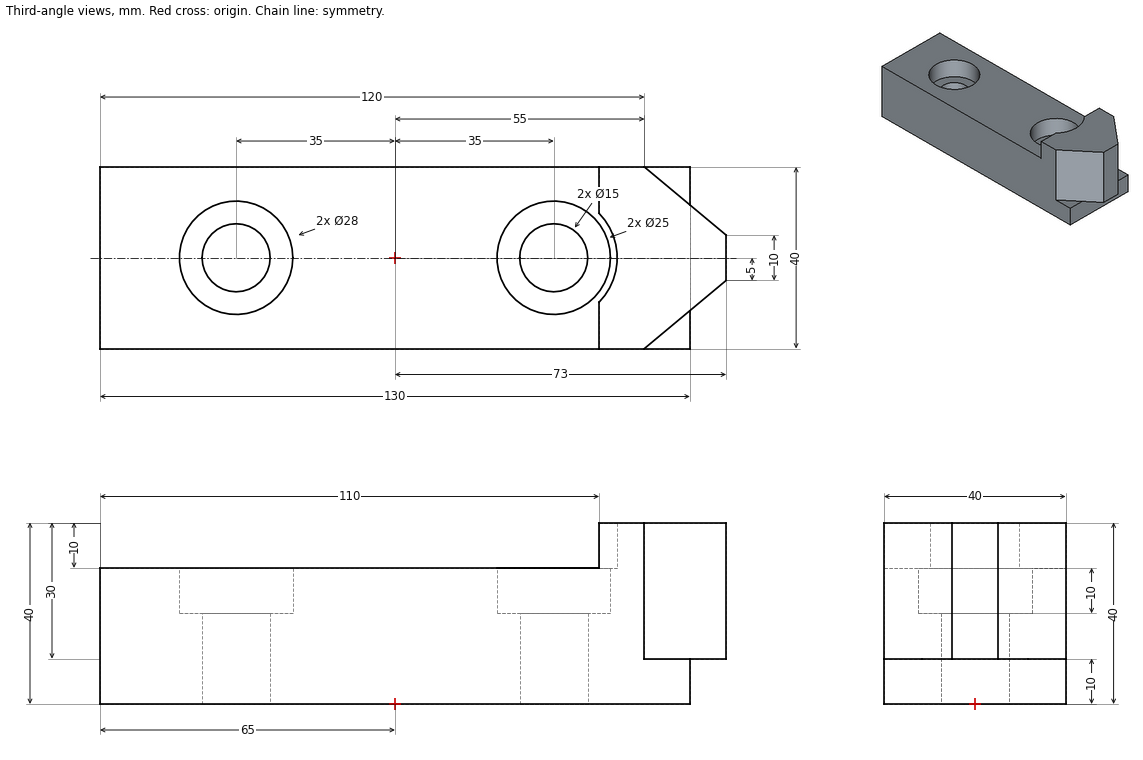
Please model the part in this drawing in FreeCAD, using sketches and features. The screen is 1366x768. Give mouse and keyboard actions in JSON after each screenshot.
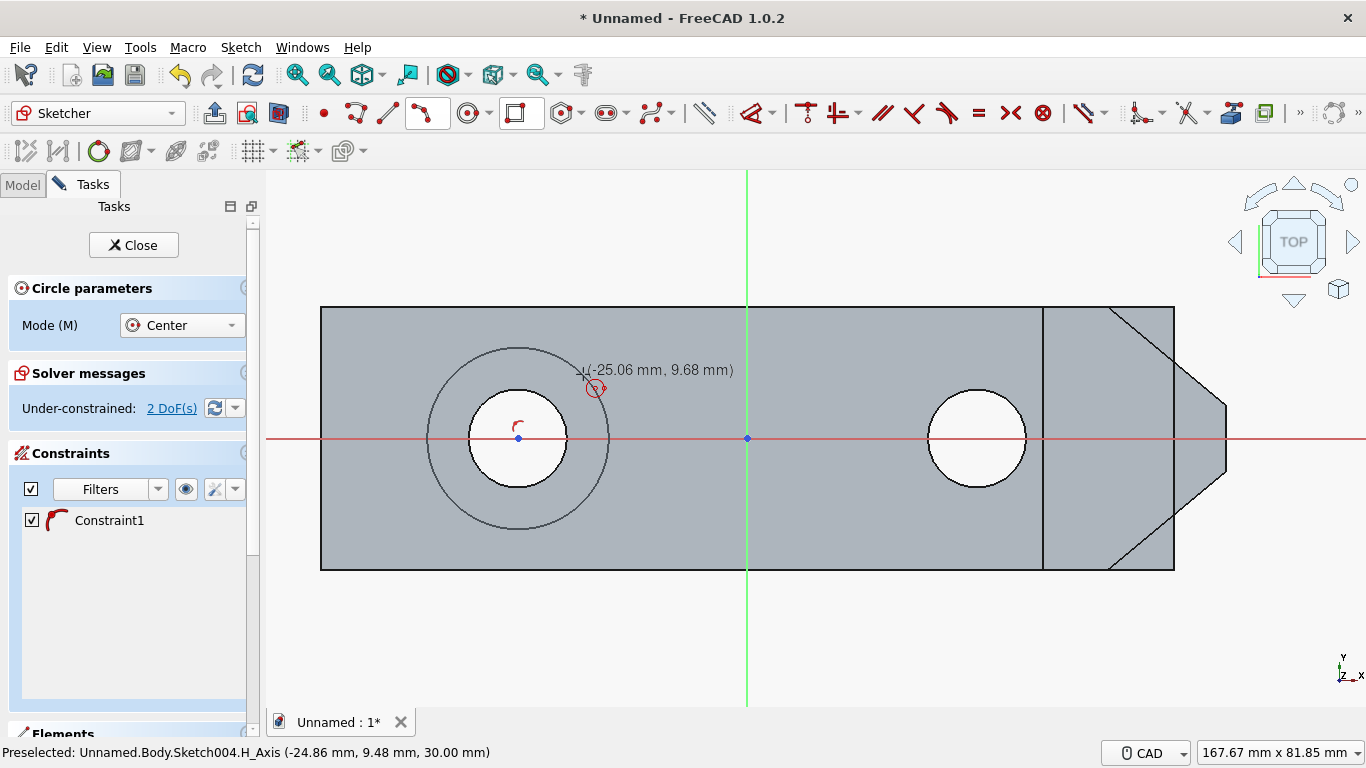
{"action": "left_click", "coordinate": [977, 438]}
{"action": "left_click", "coordinate": [1042, 374]}
{"action": "key", "text": "Escape"}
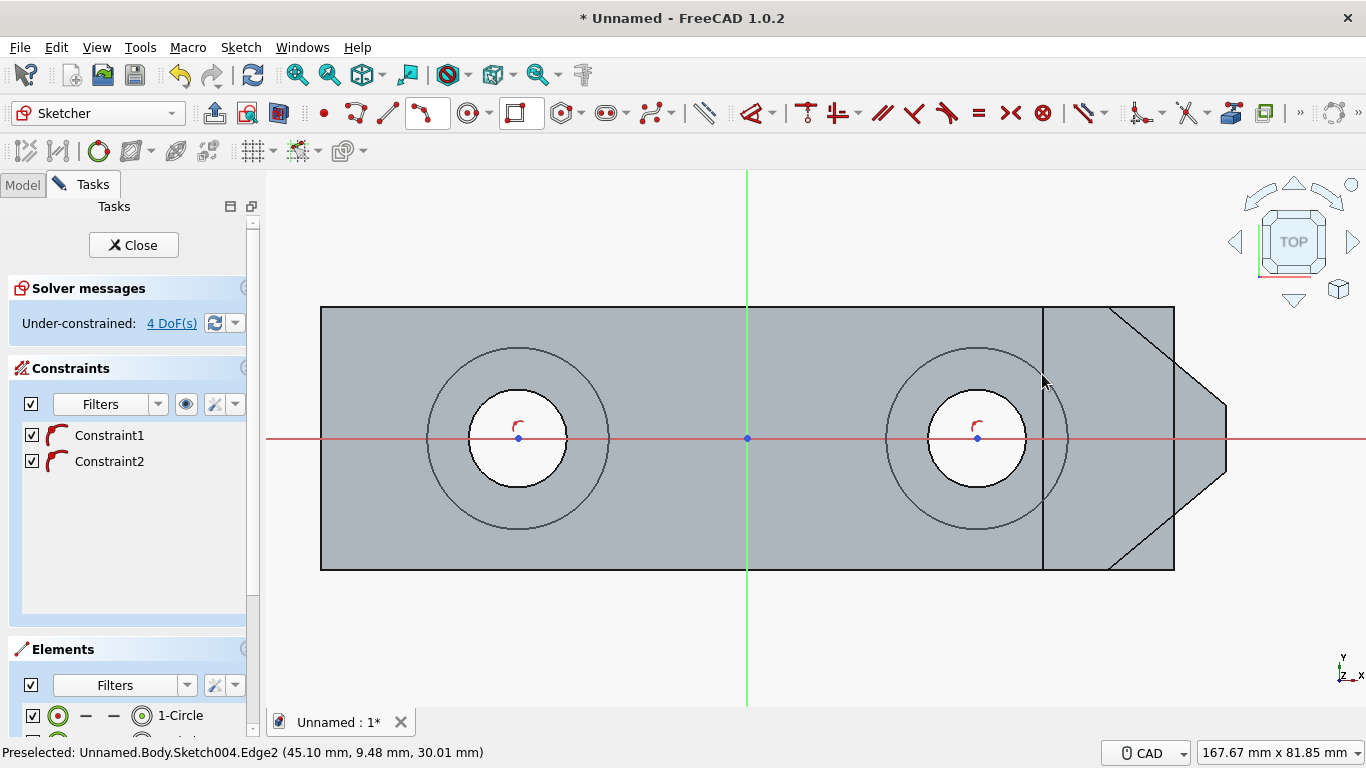
{"action": "left_click", "coordinate": [582, 374]}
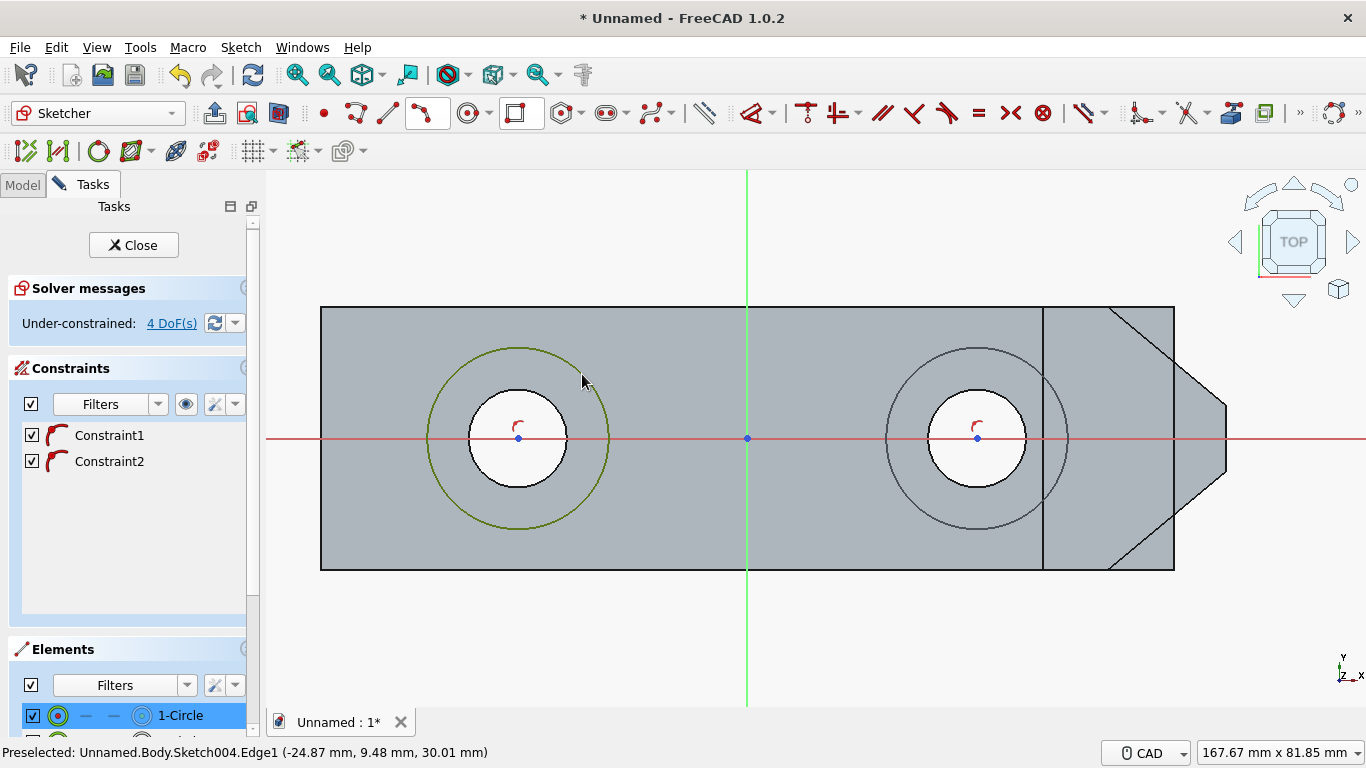
{"action": "left_click", "coordinate": [1041, 374]}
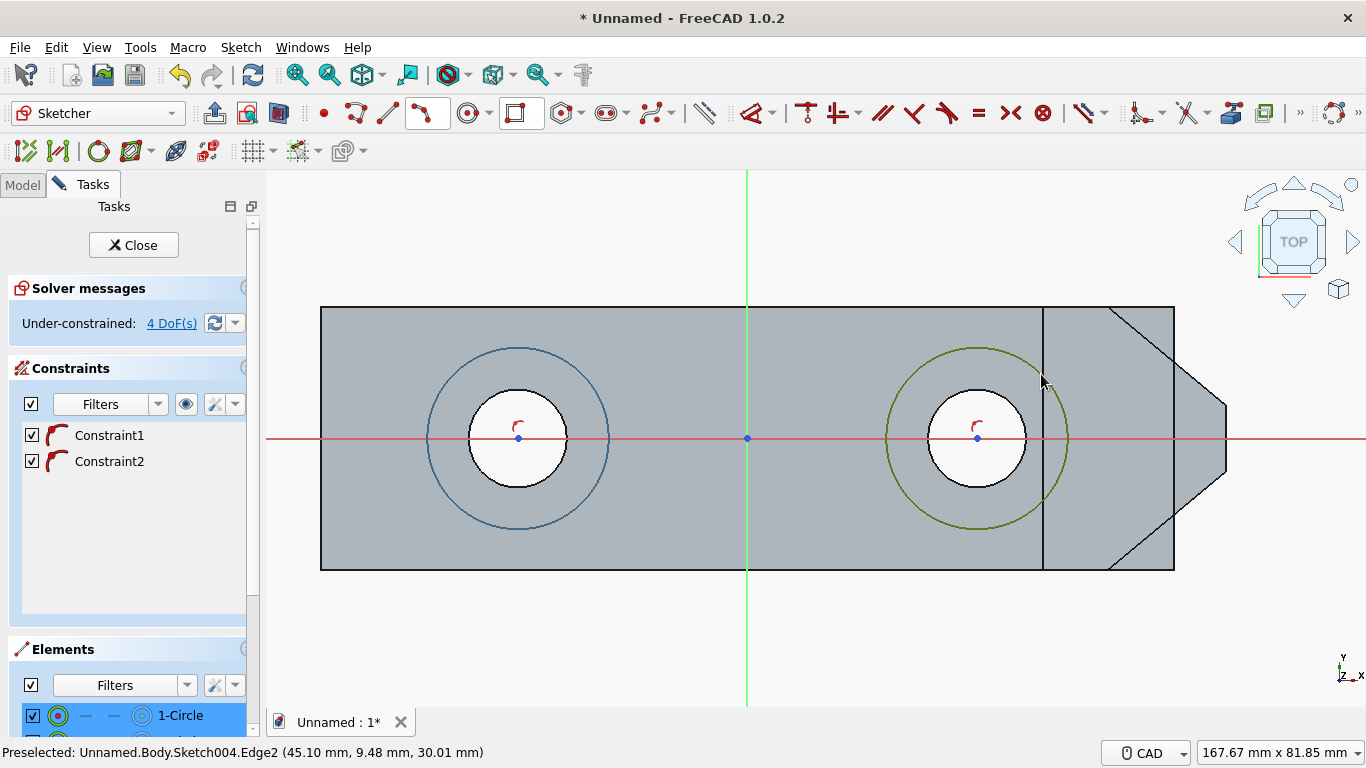
{"action": "key", "text": "e"}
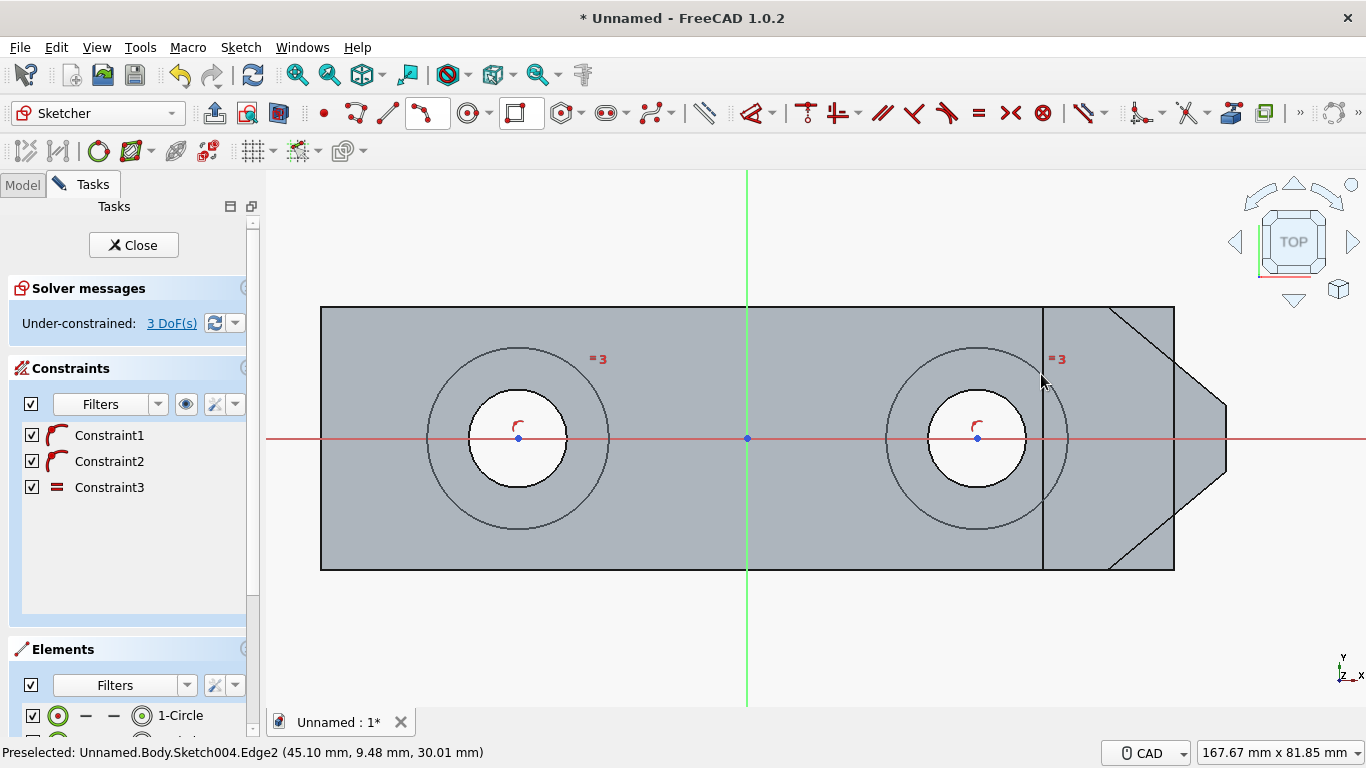
{"action": "left_click", "coordinate": [752, 114]}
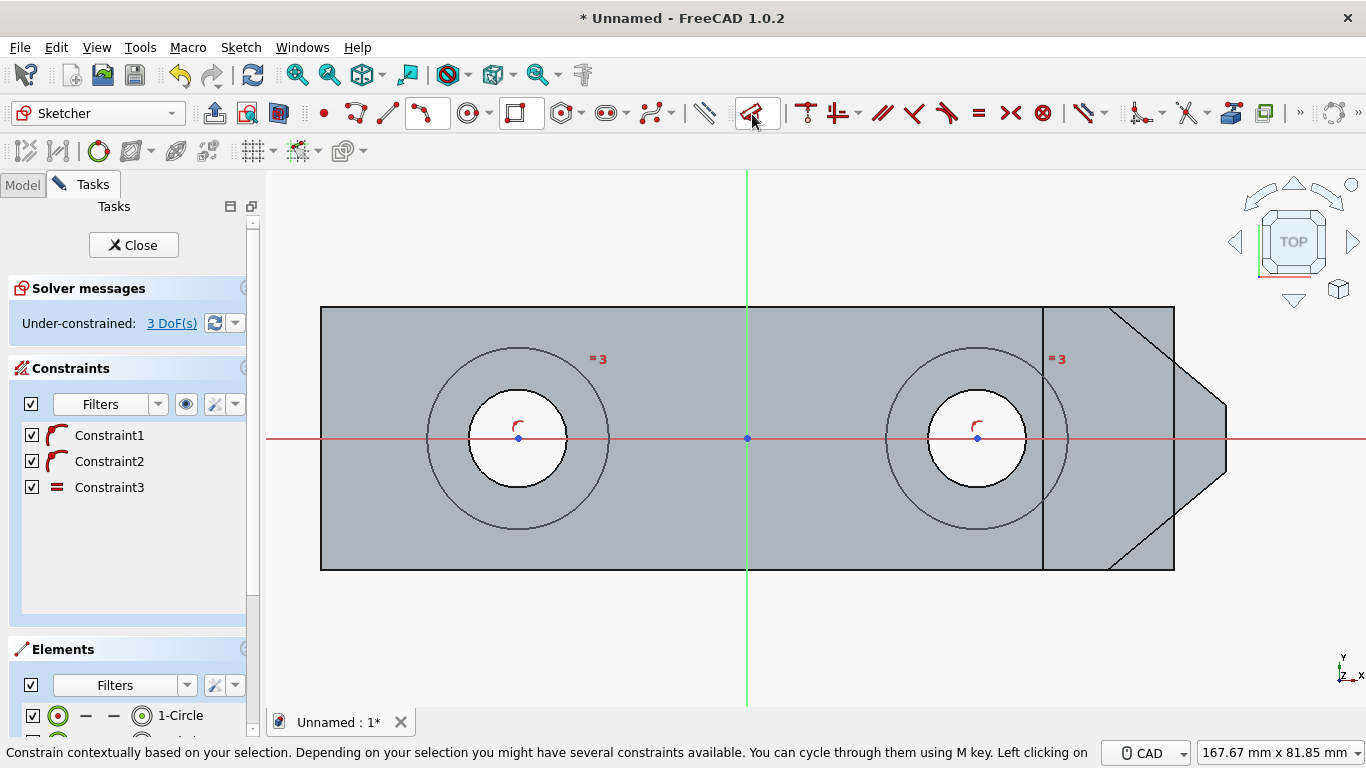
{"action": "left_click", "coordinate": [582, 374]}
{"action": "left_click", "coordinate": [605, 351]}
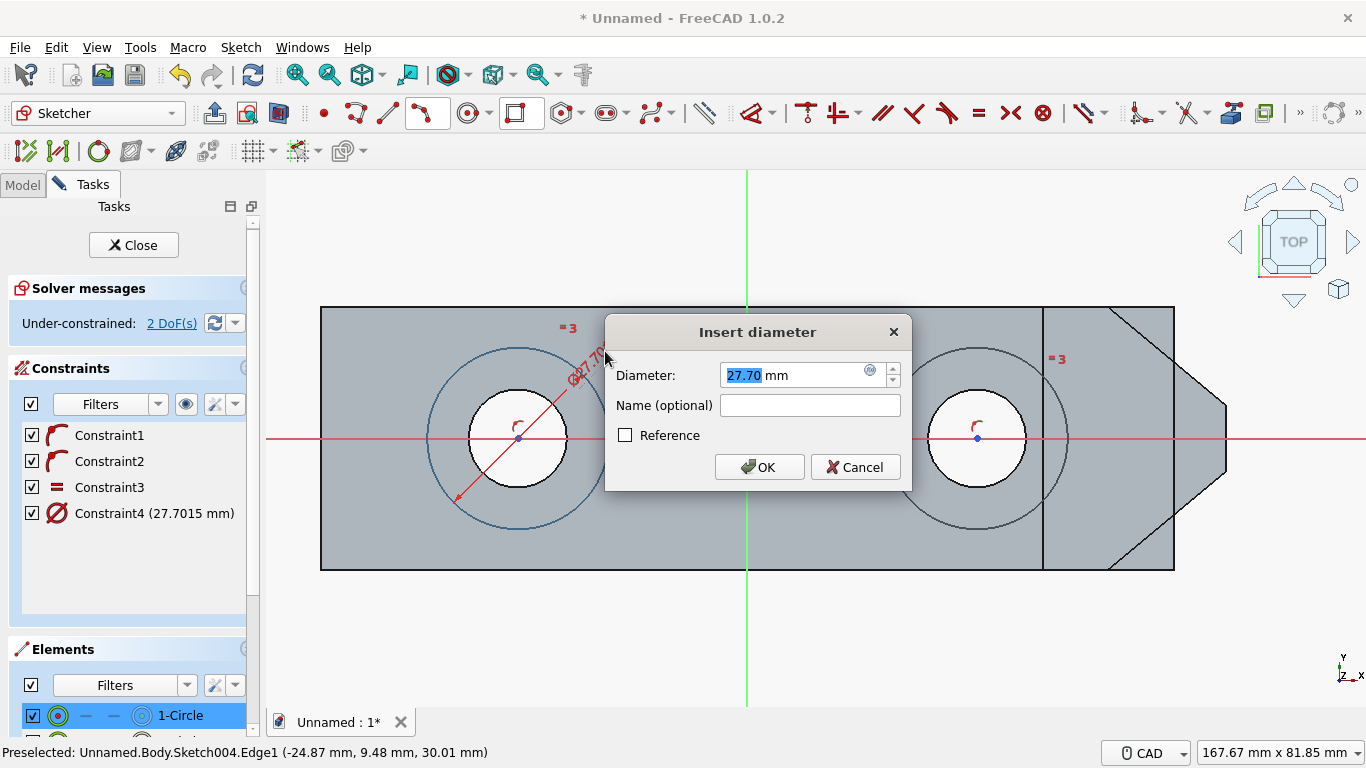
{"action": "type", "text": "28"}
{"action": "key", "text": "Return"}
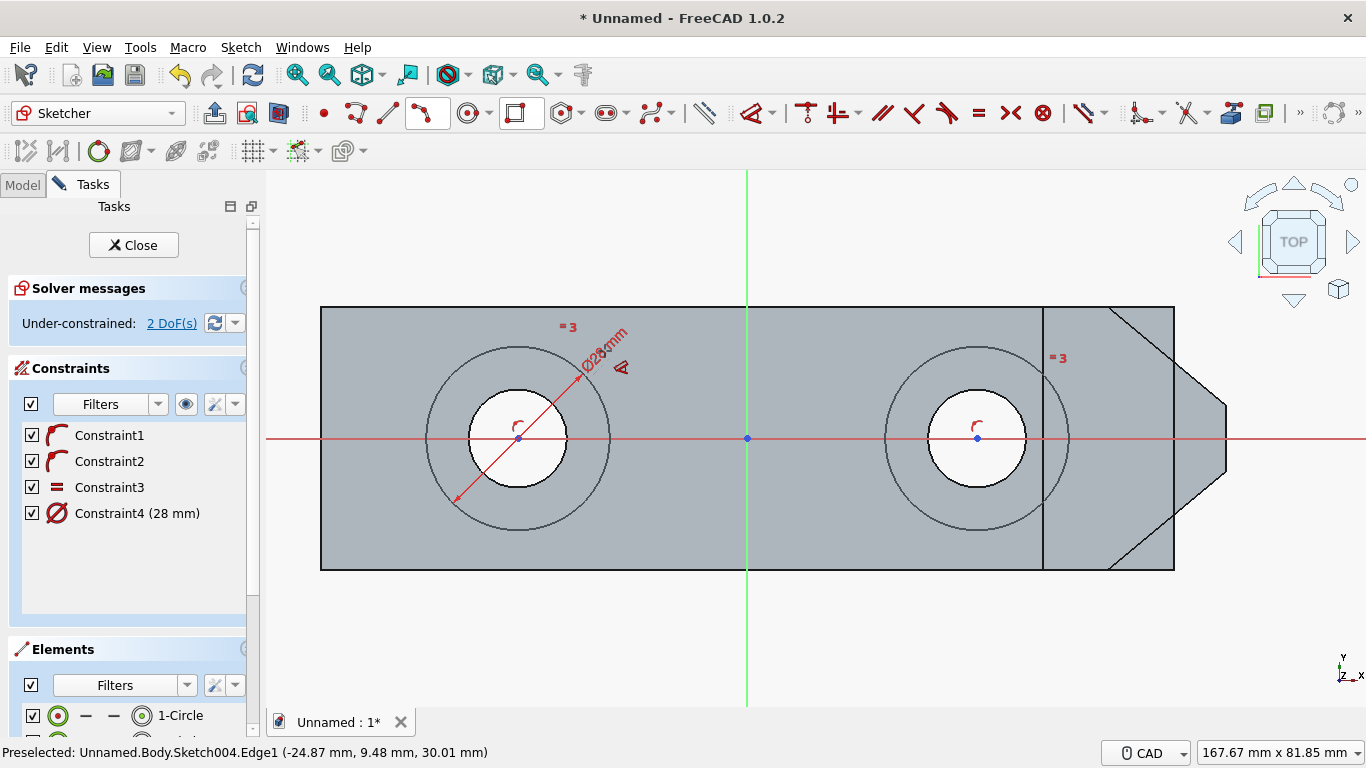
{"action": "left_click", "coordinate": [518, 438]}
{"action": "left_click", "coordinate": [633, 472]}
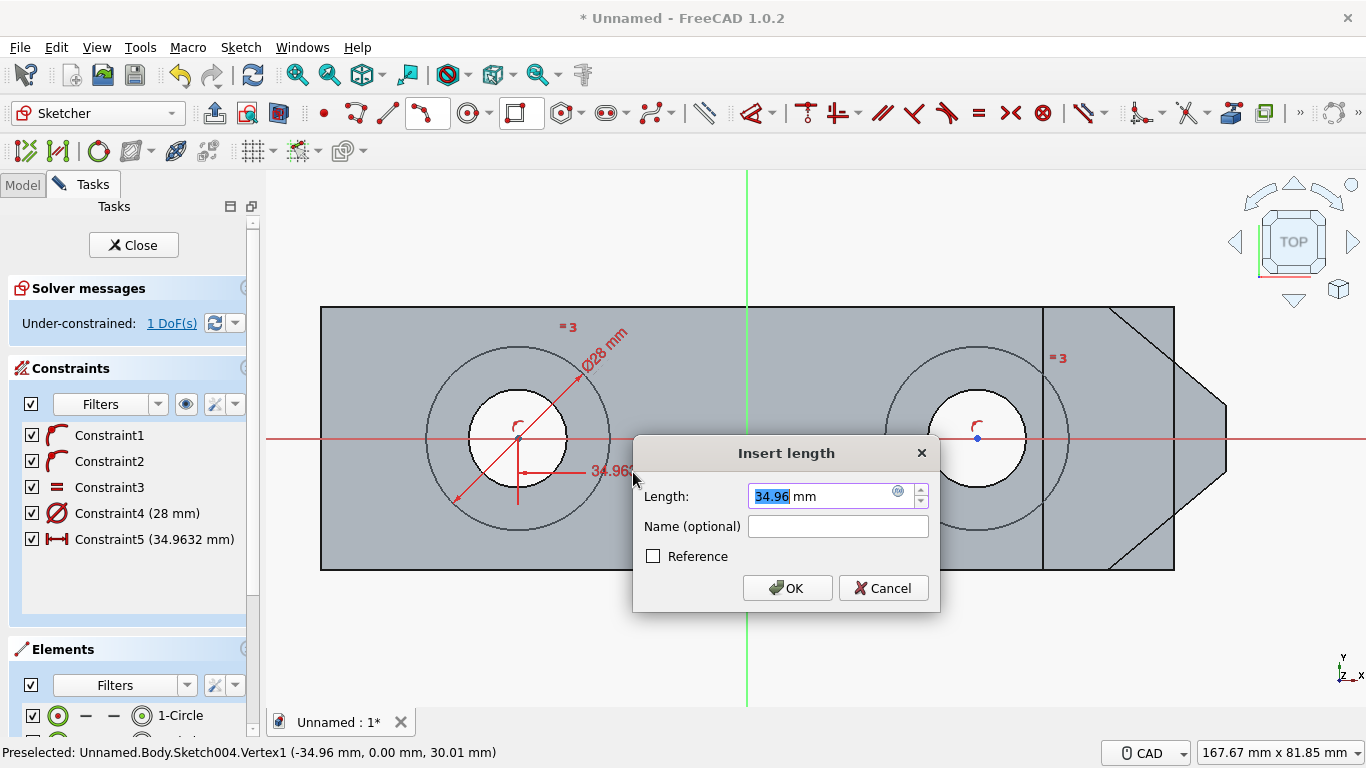
{"action": "type", "text": "35"}
{"action": "key", "text": "Return"}